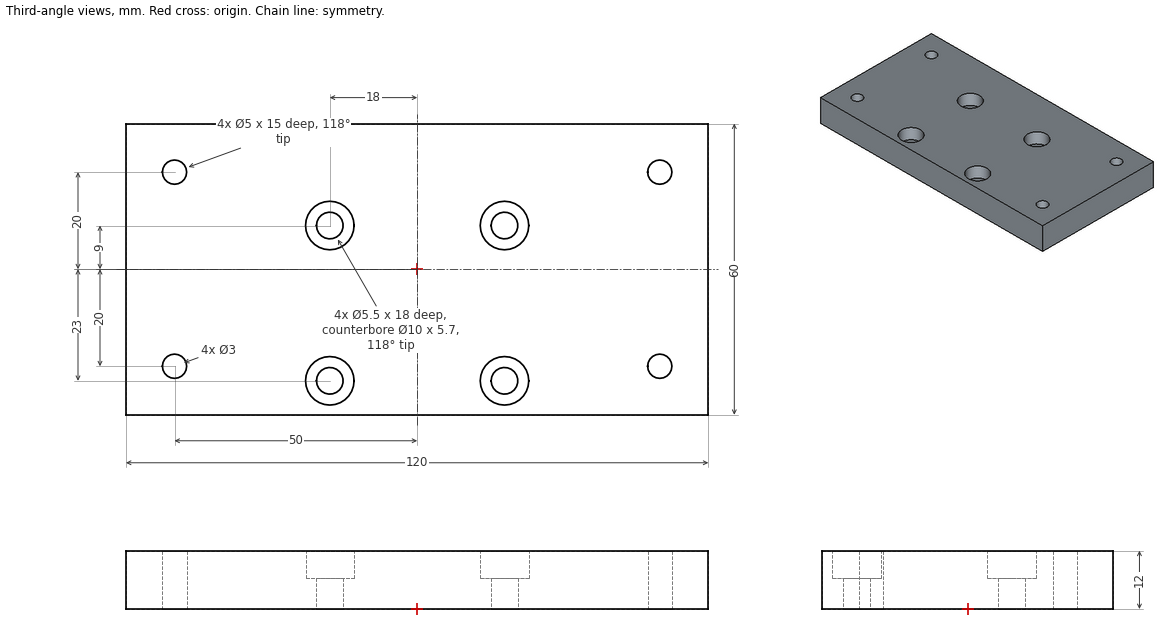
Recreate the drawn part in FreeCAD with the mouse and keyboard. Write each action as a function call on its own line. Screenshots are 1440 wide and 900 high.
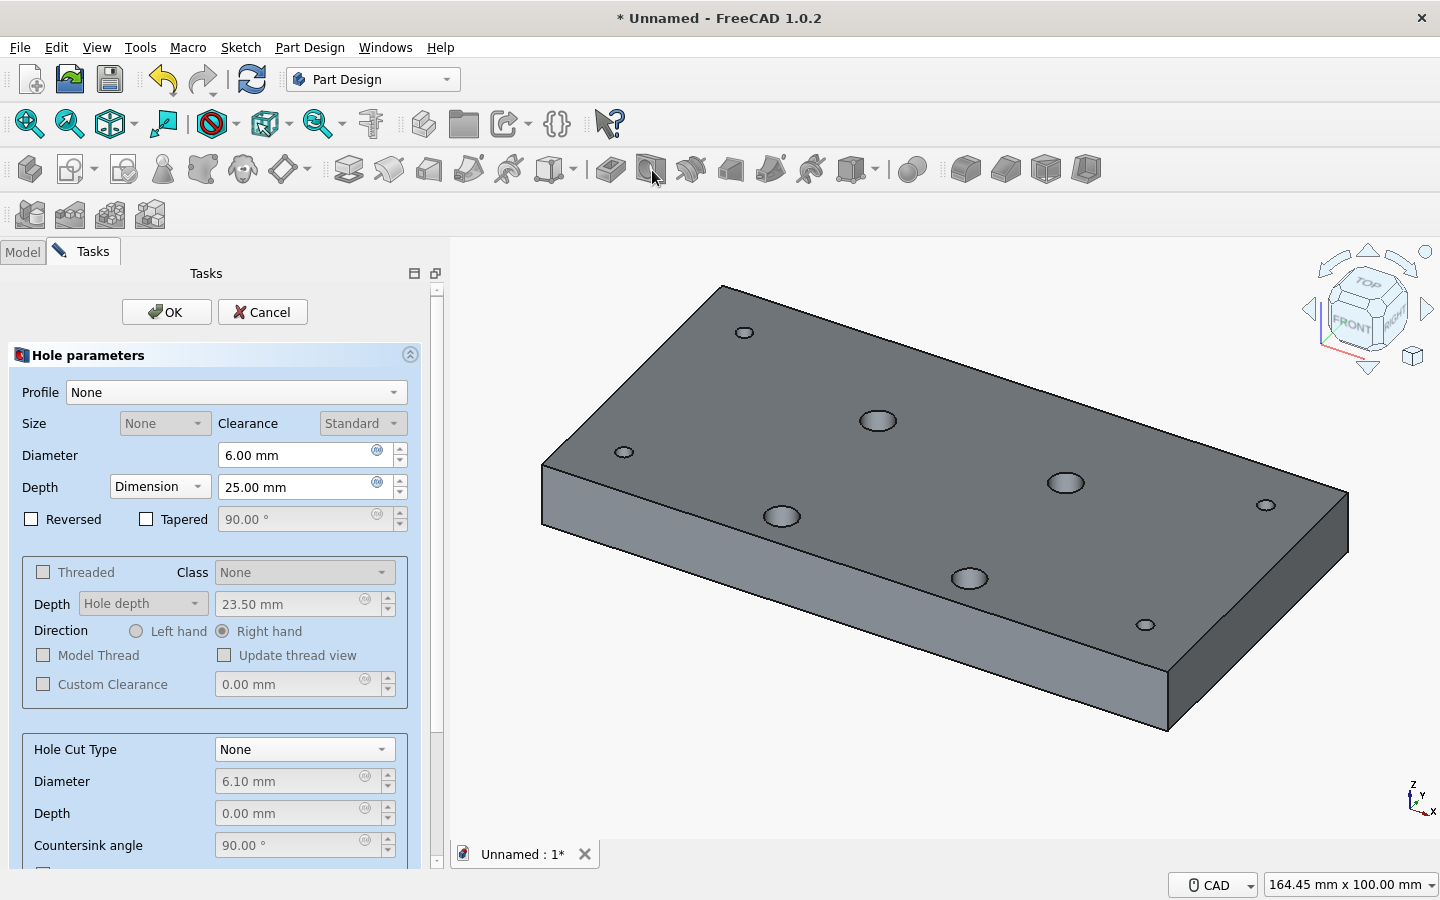
triple_click(305, 455)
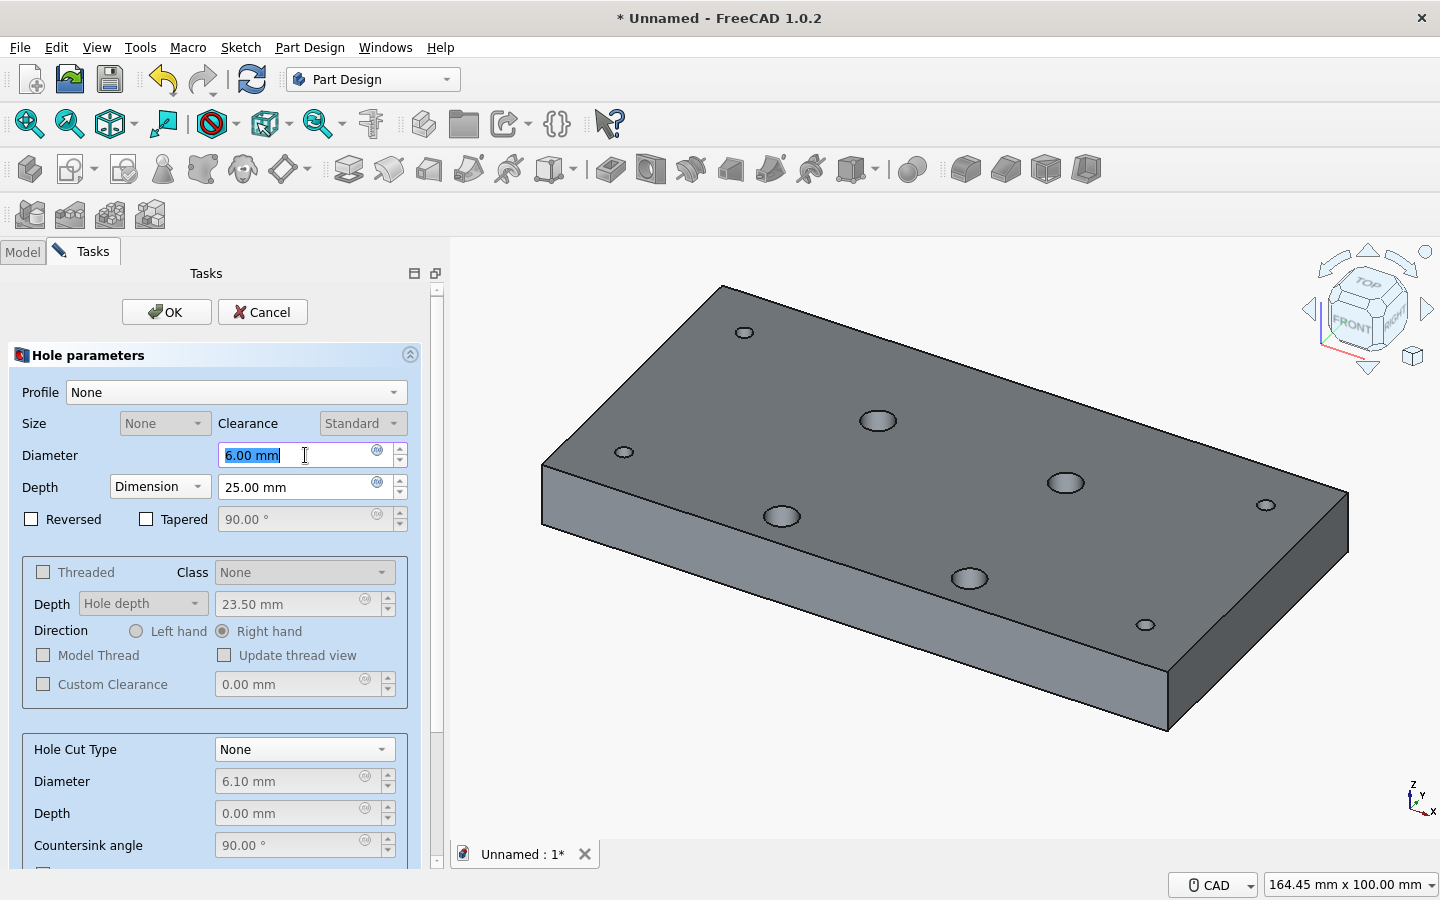
text(5.5)
key(Tab)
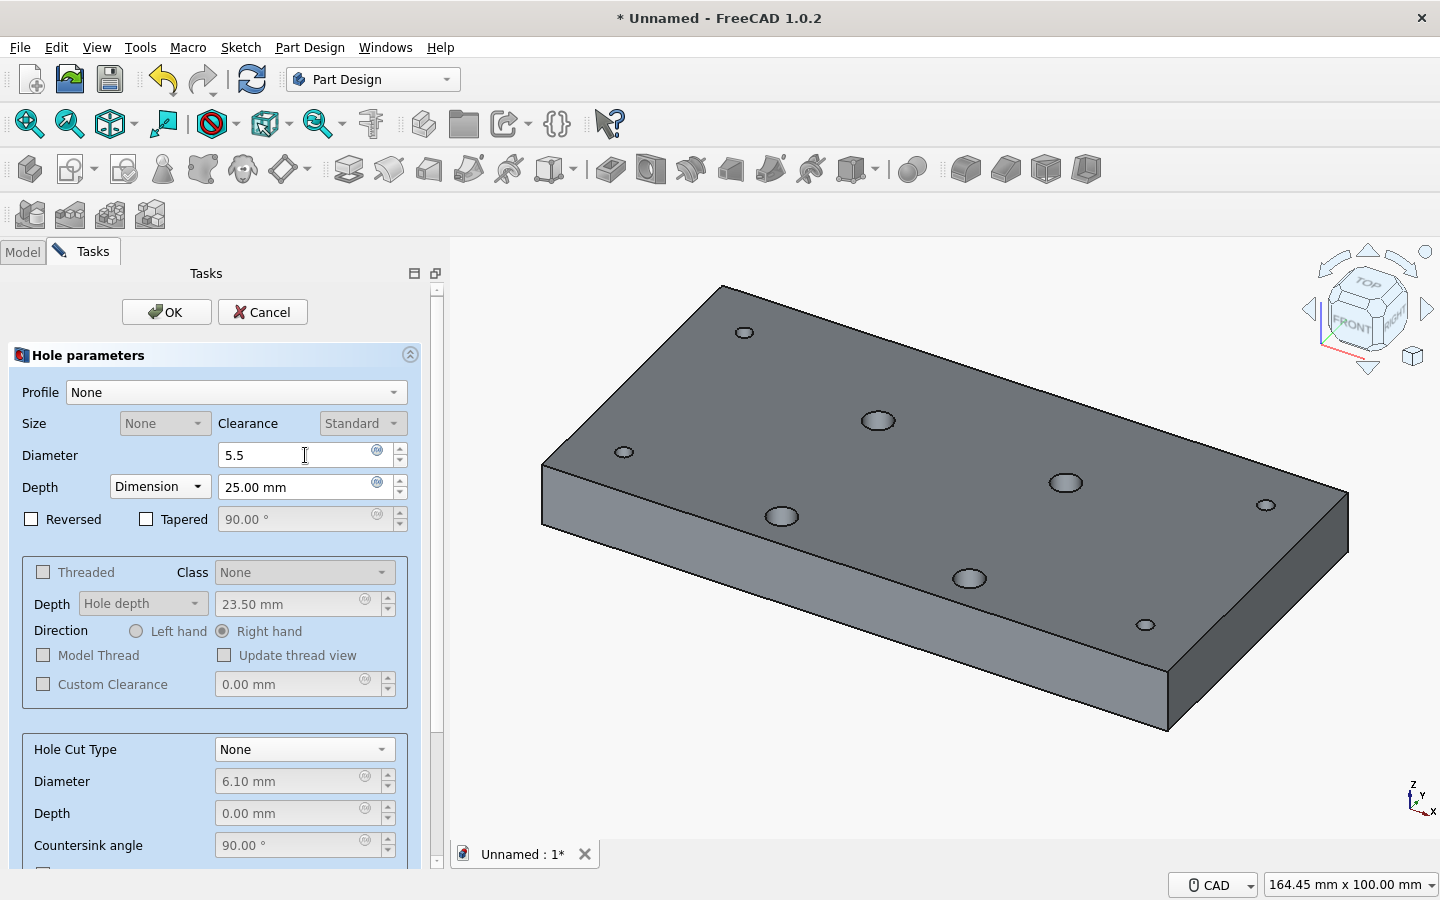
triple_click(305, 487)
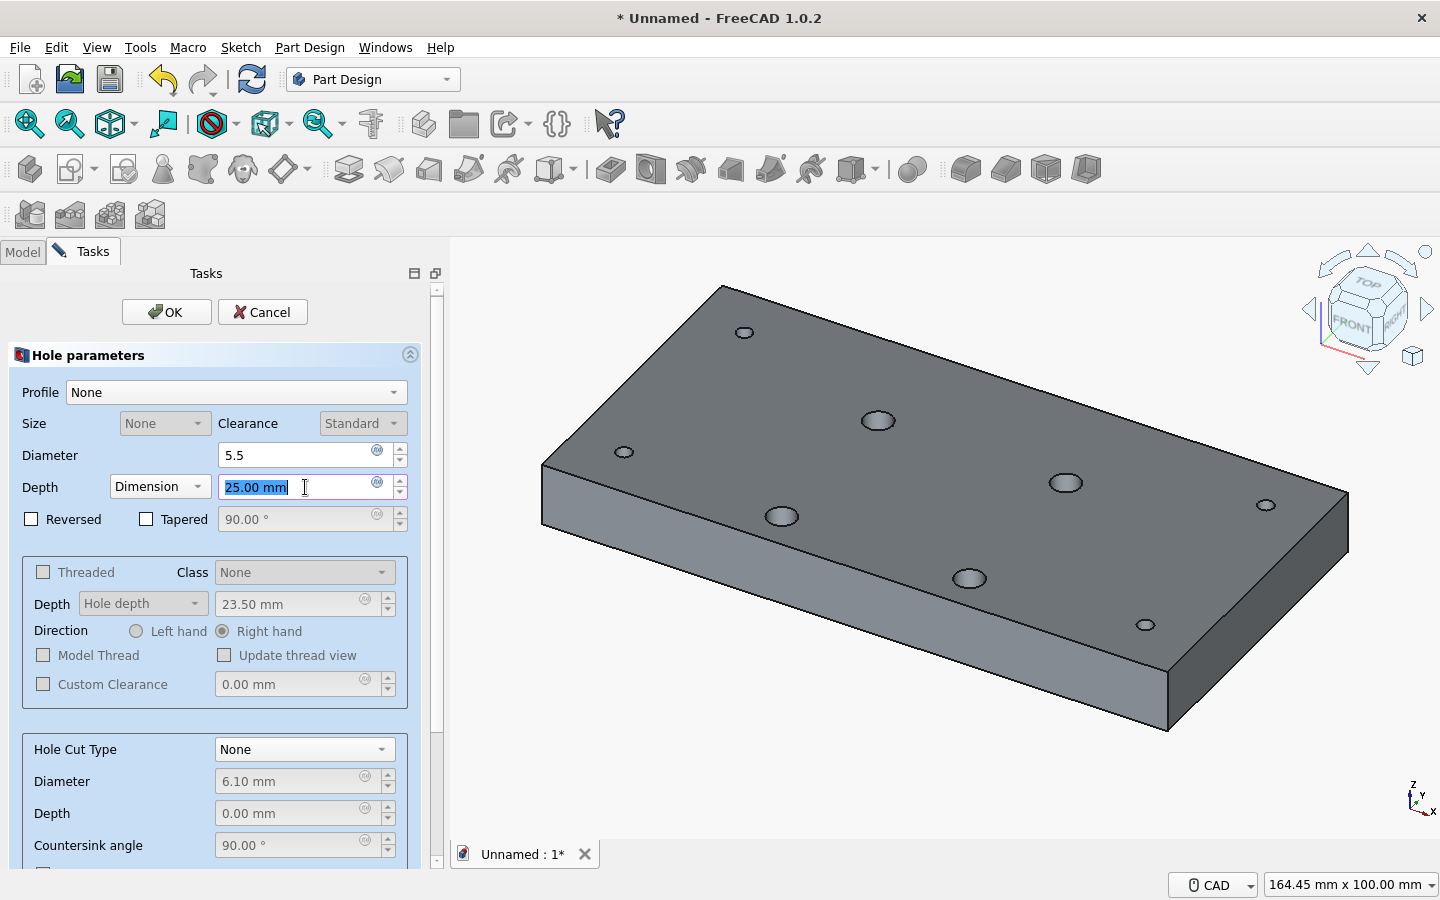
text(18)
key(Tab)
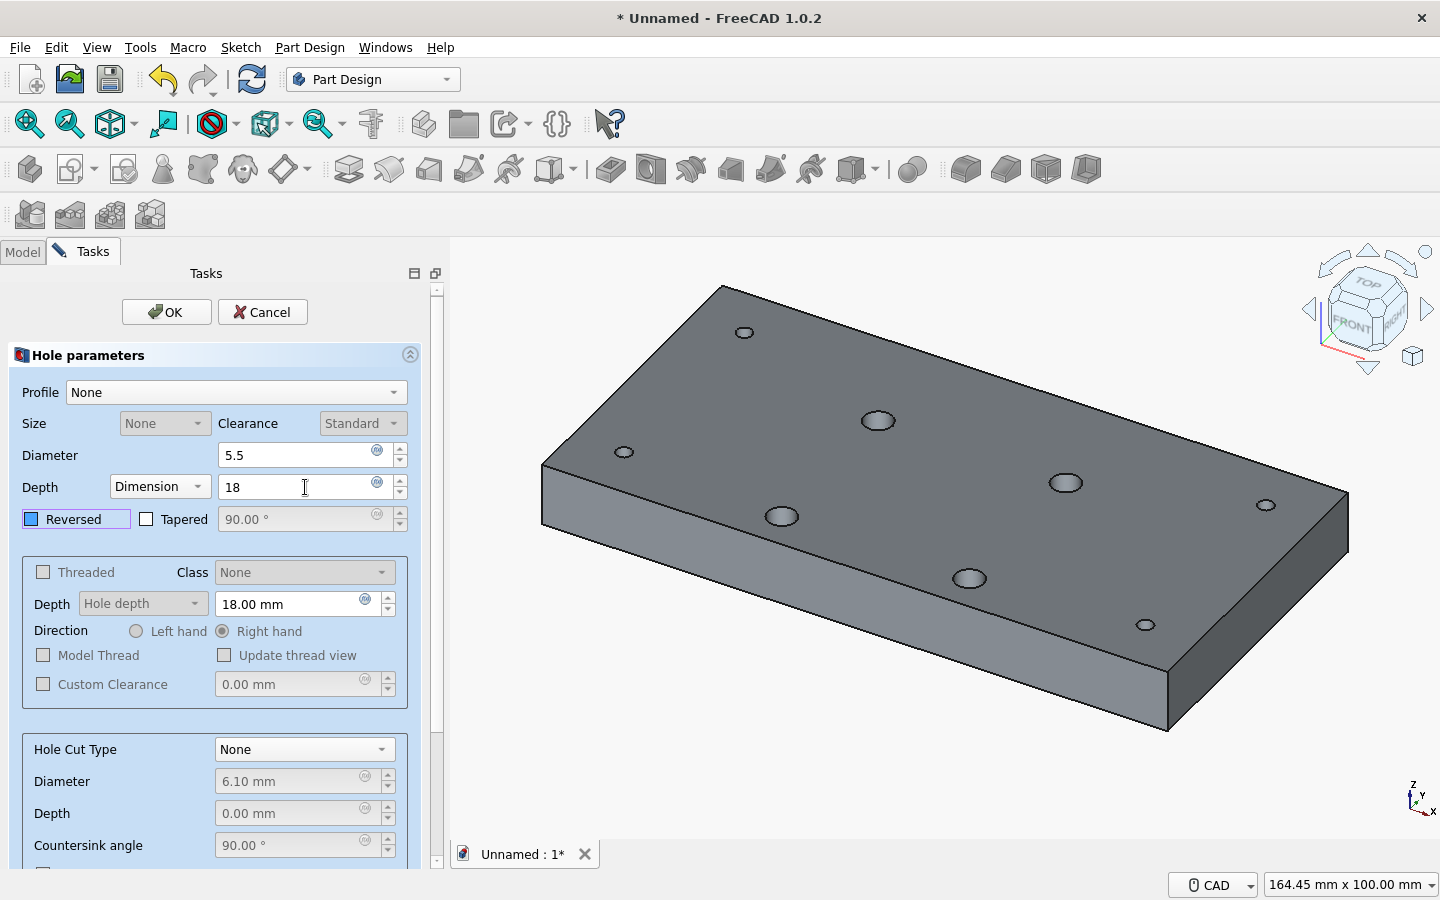
click(306, 750)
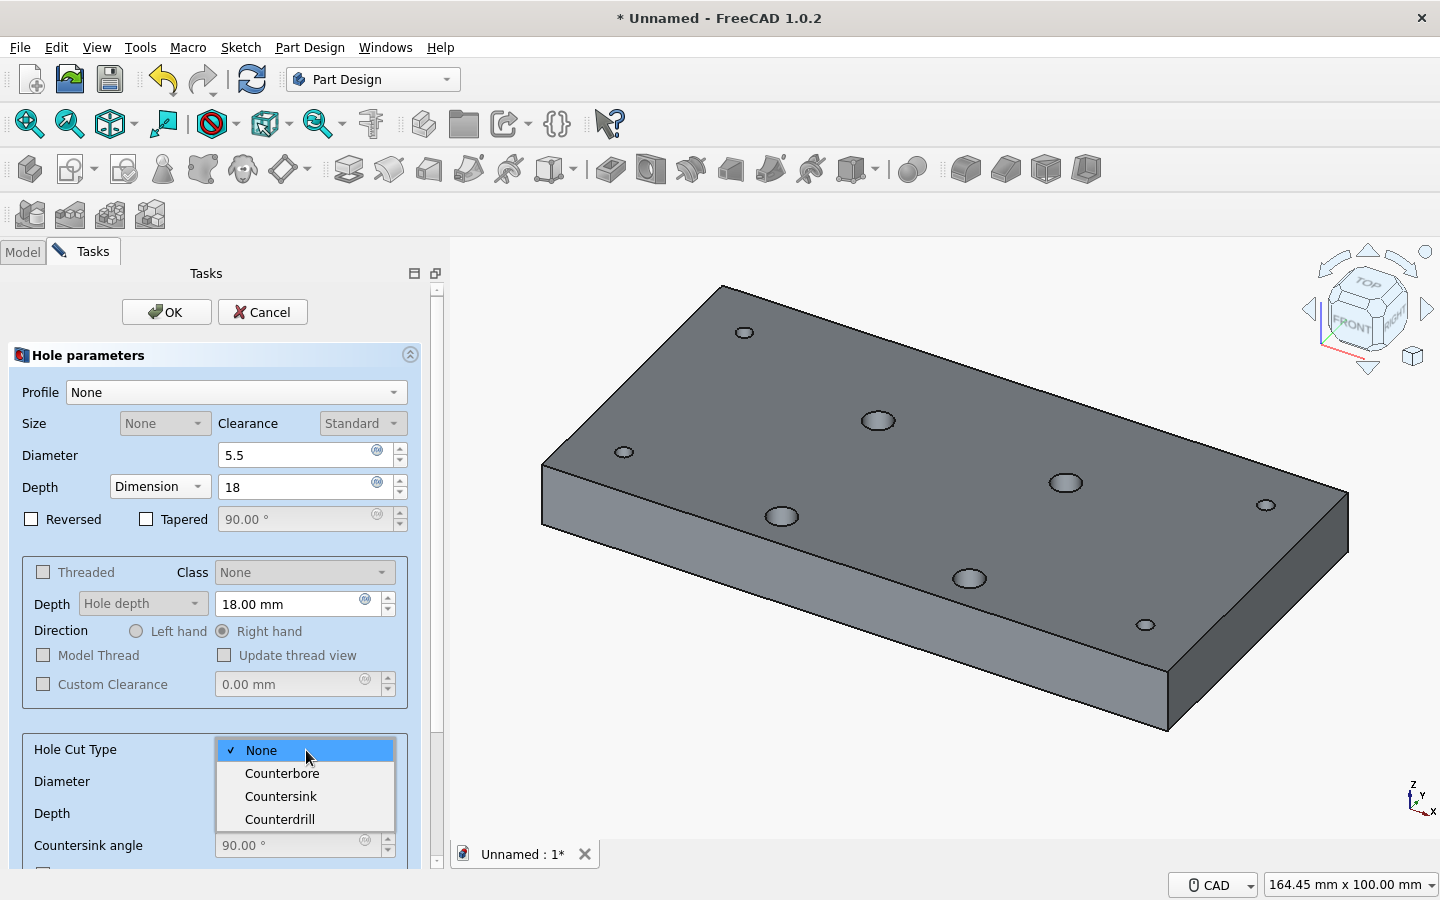
click(304, 774)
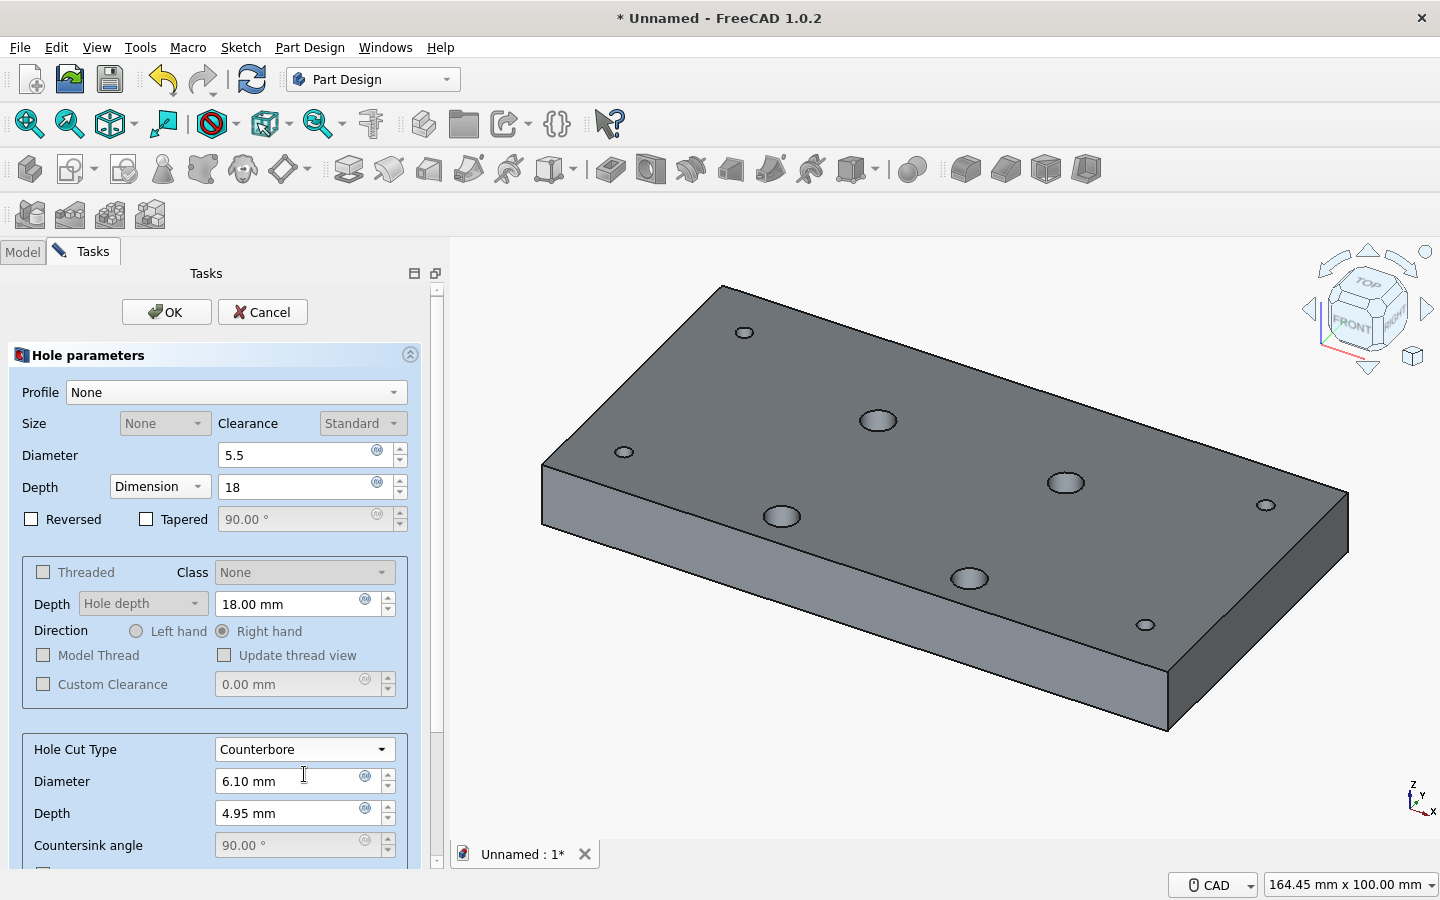
triple_click(298, 781)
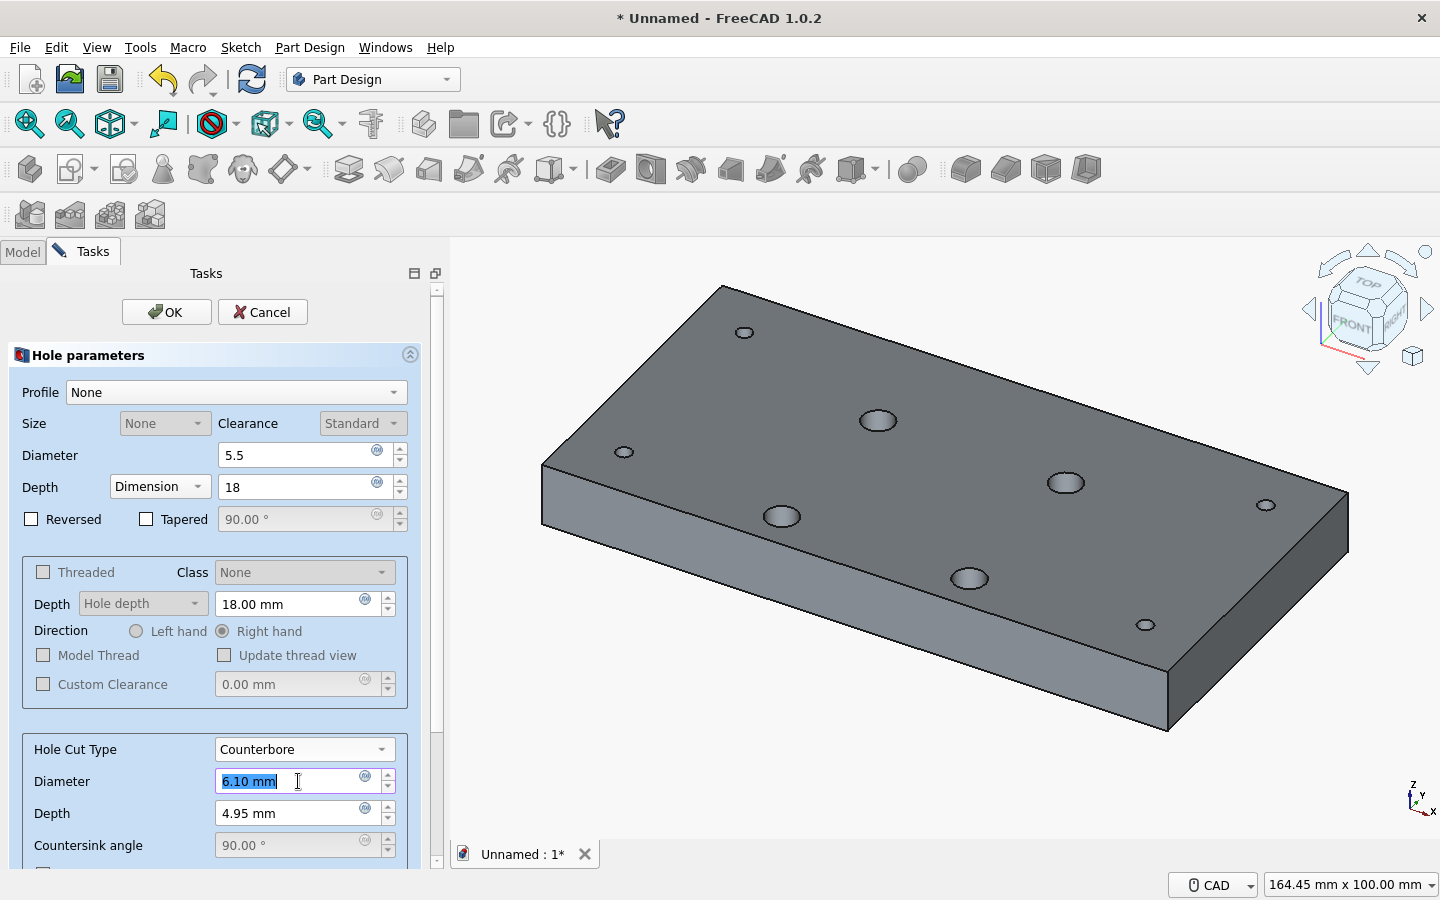
text(10)
key(Tab)